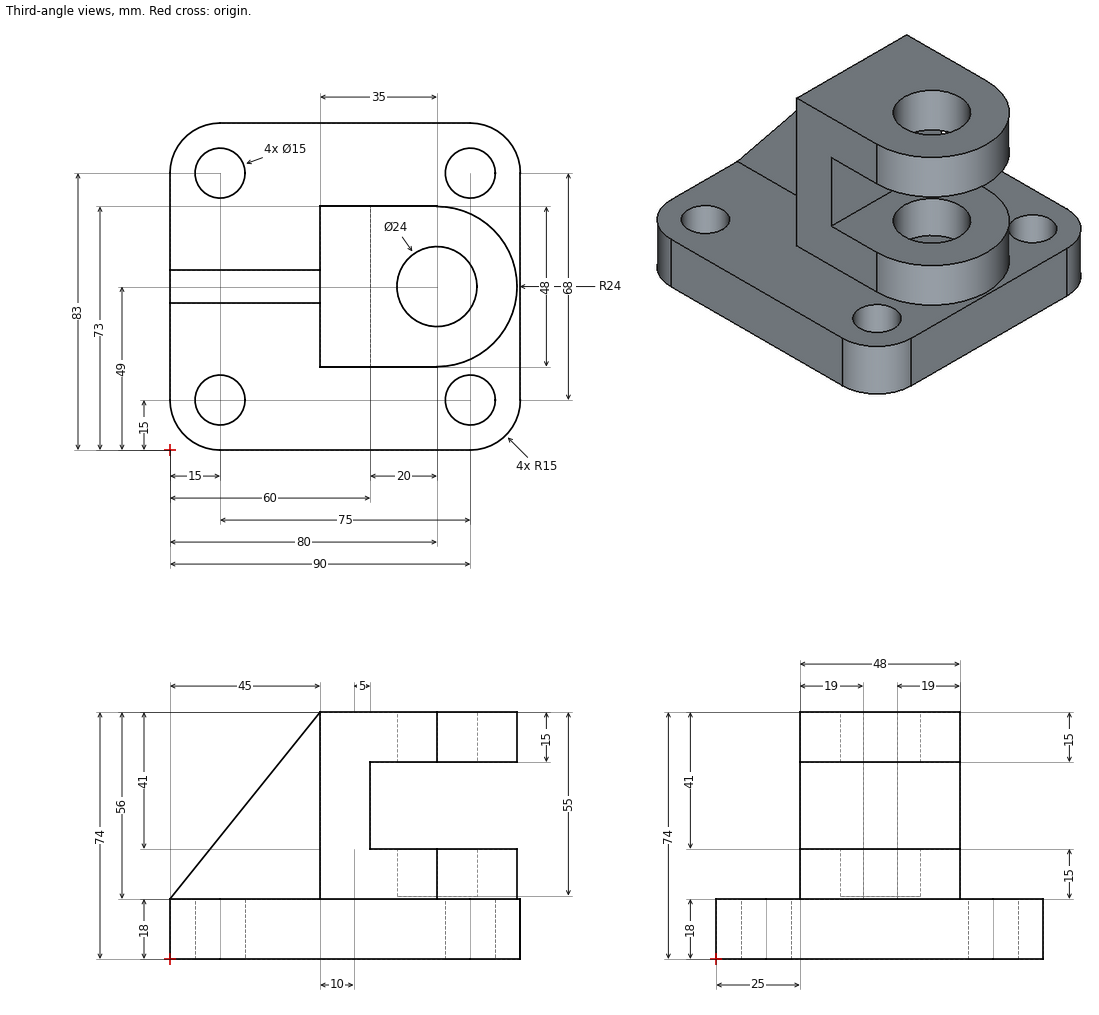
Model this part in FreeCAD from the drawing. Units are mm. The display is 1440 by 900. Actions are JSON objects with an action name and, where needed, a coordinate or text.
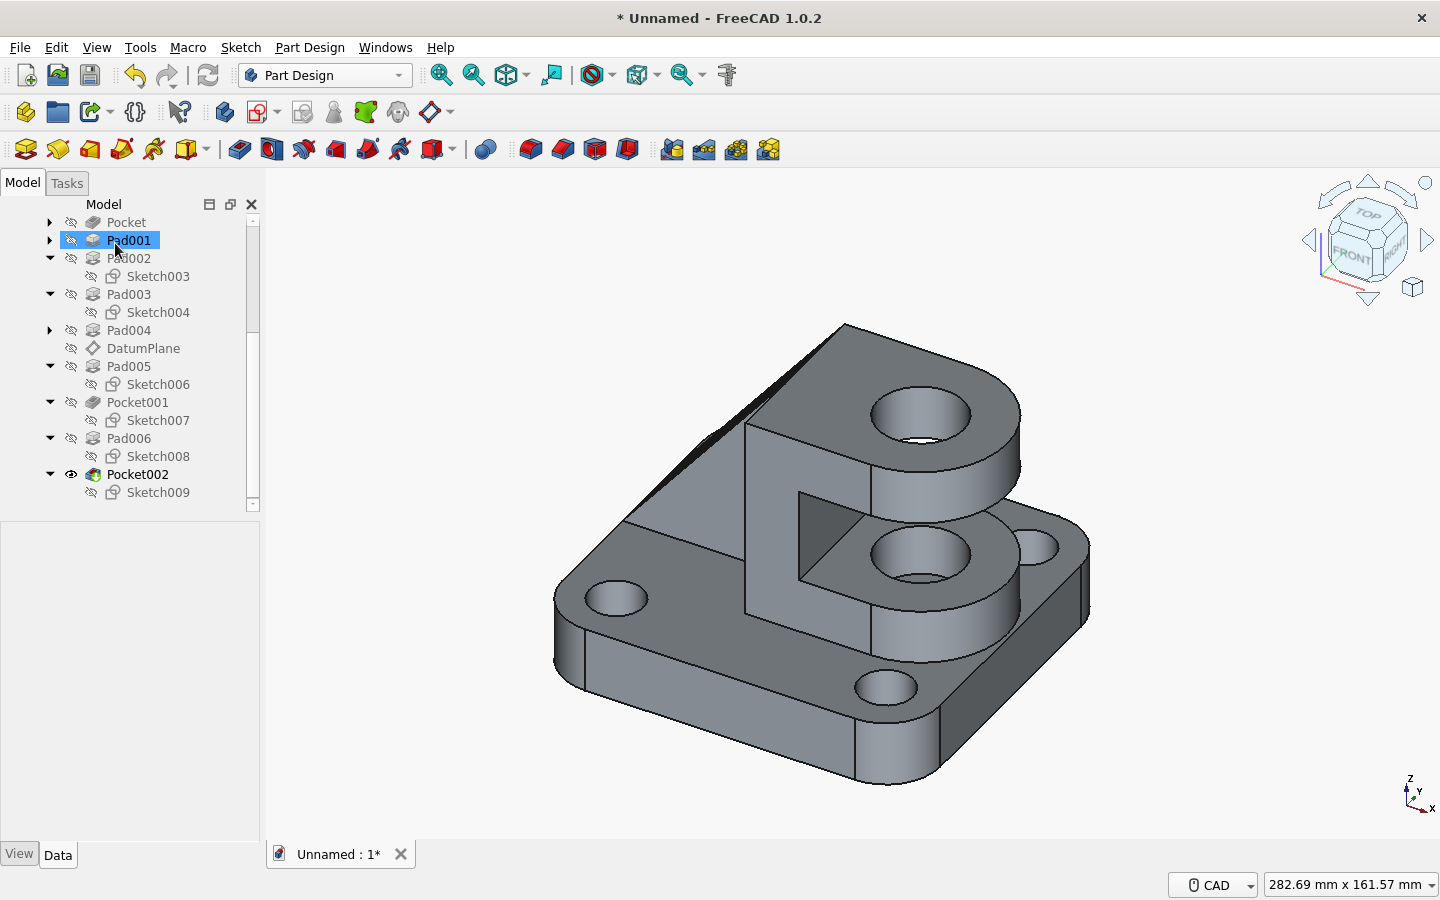
{"action": "key", "text": "4"}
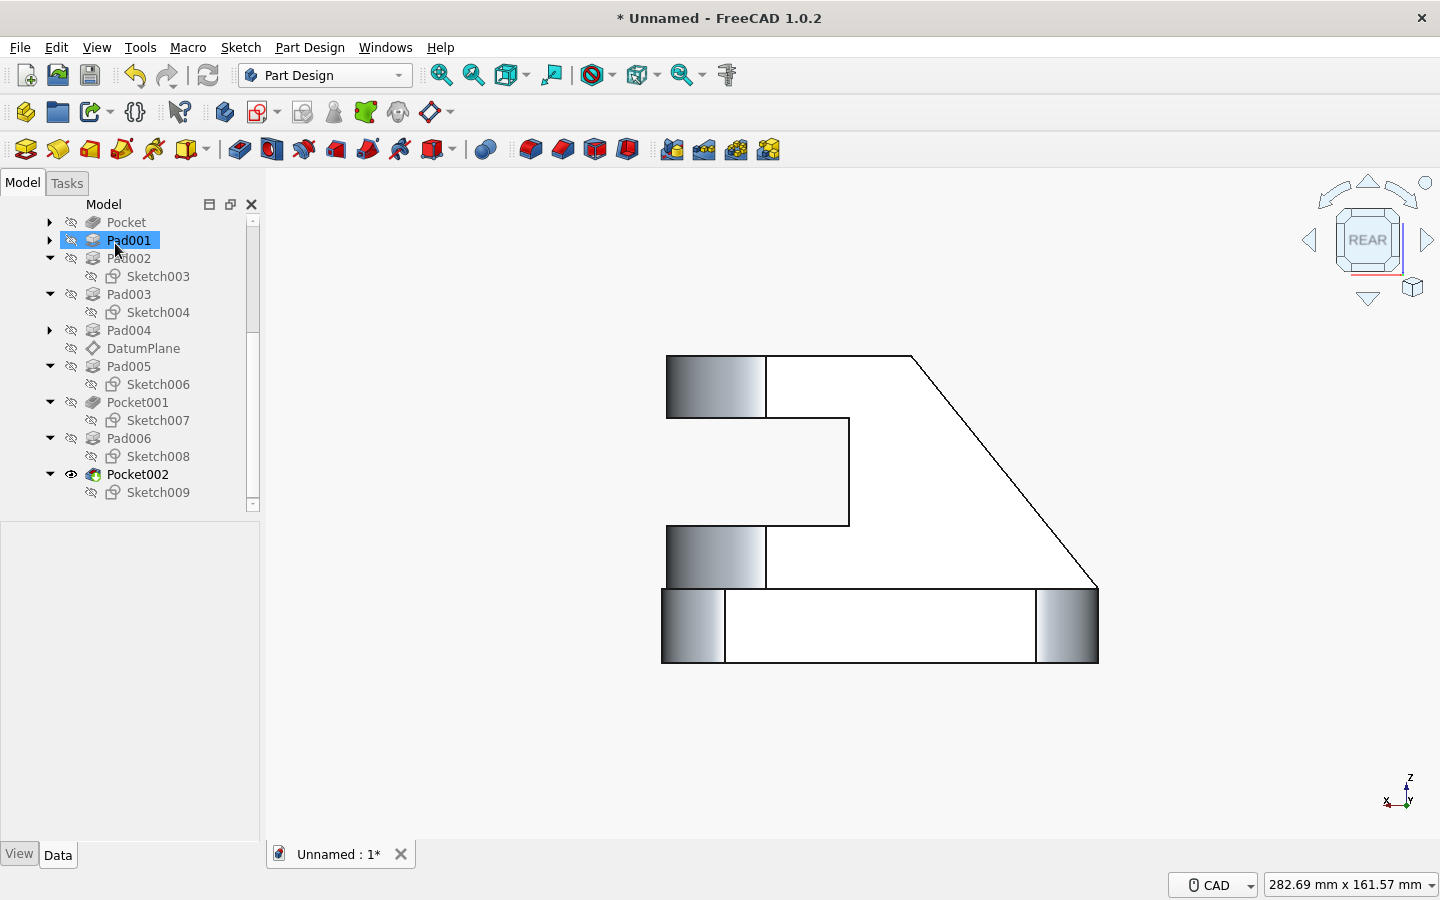
{"action": "left_click", "coordinate": [932, 505]}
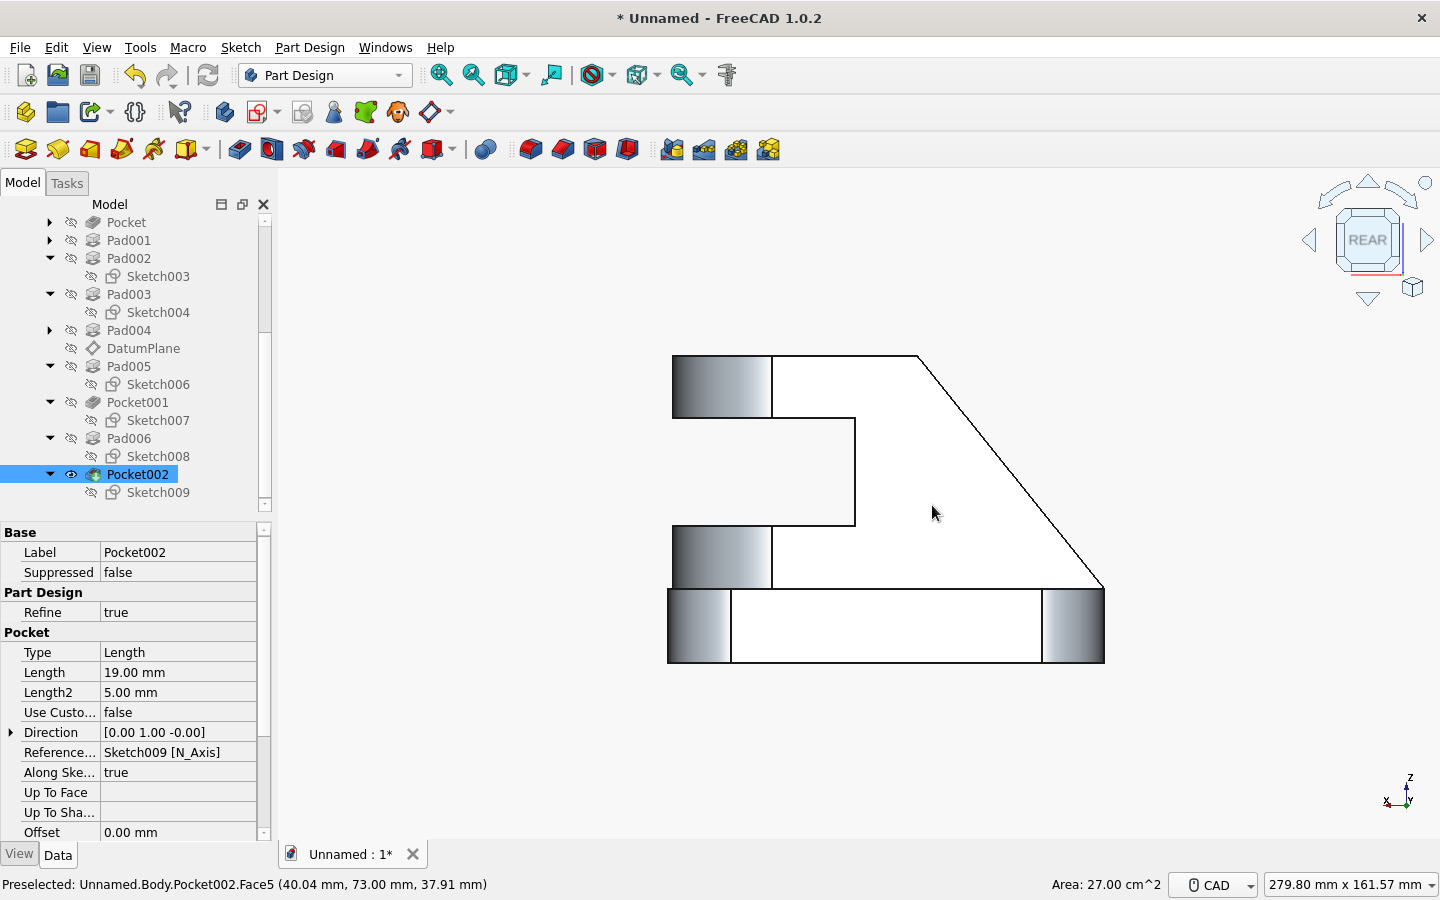
{"action": "left_click", "coordinate": [258, 112]}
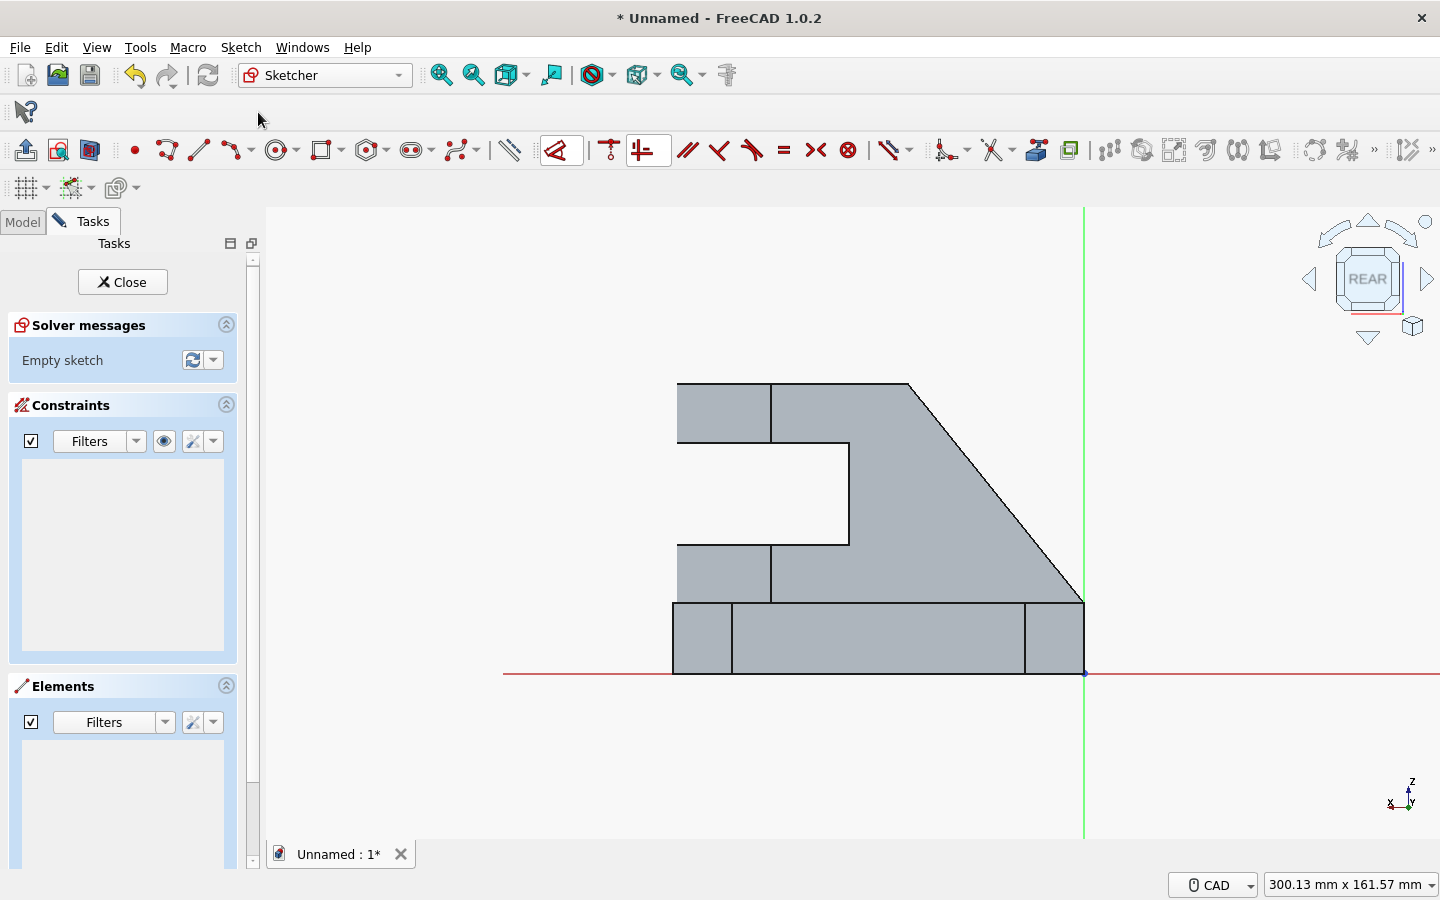
{"action": "left_click", "coordinate": [90, 150]}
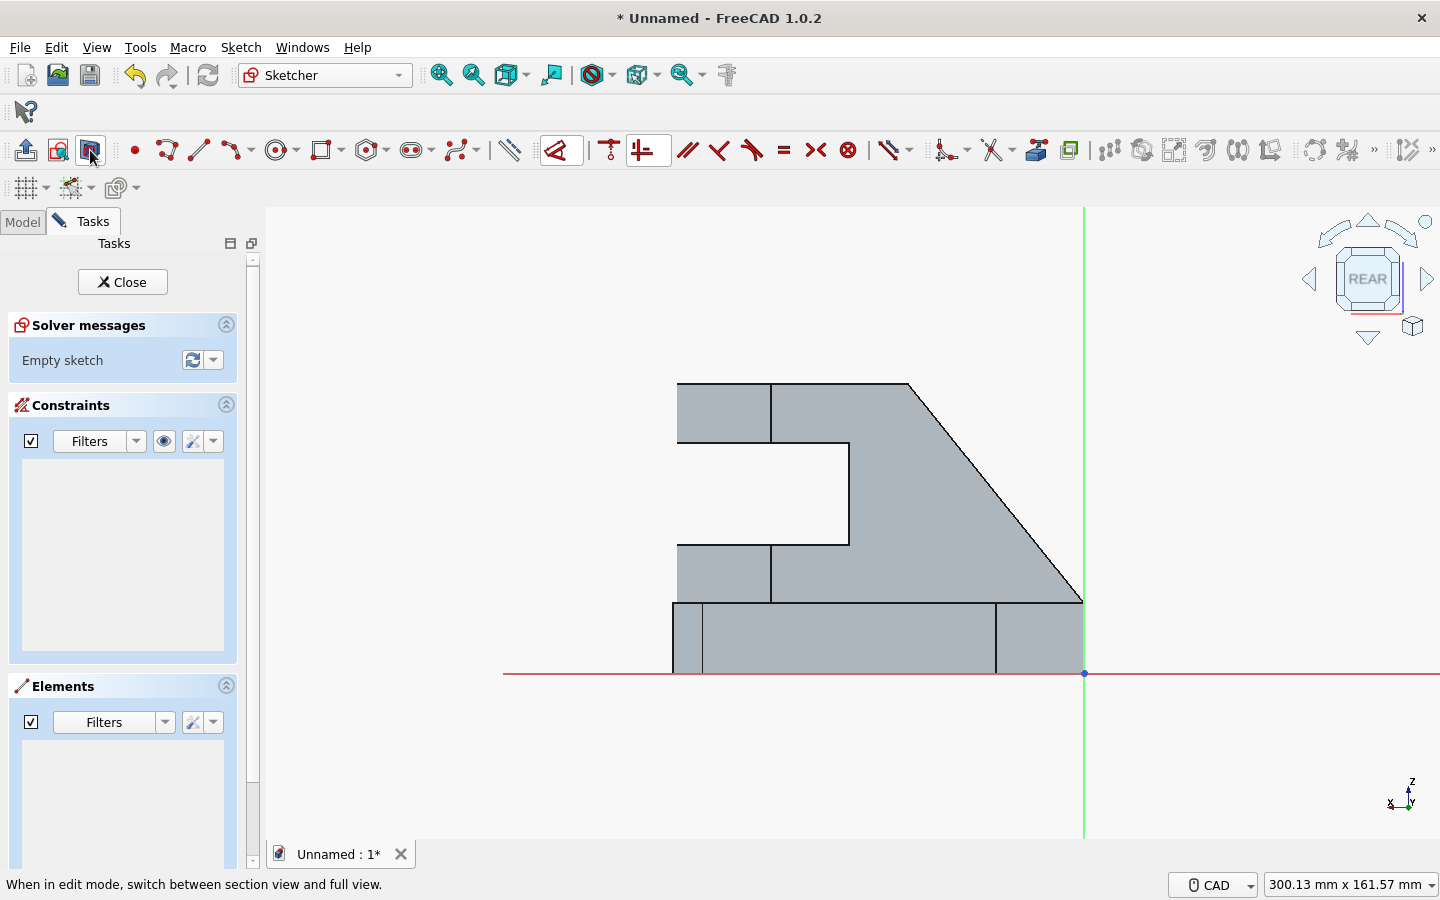
{"action": "scroll", "coordinate": [1275, 541], "scroll_direction": "up", "scroll_amount": 2}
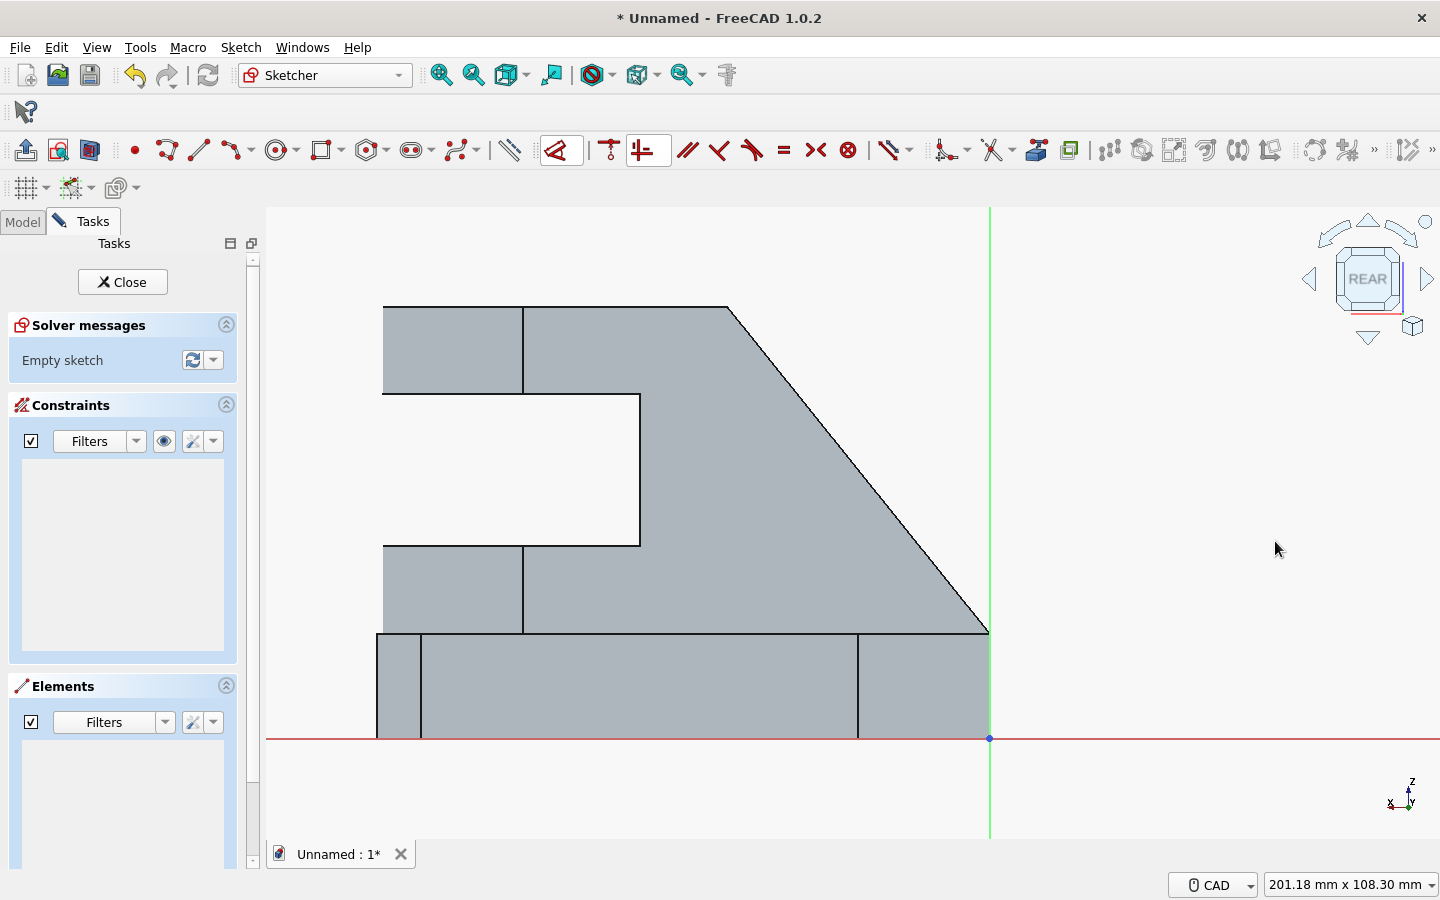
{"action": "left_click", "coordinate": [168, 150]}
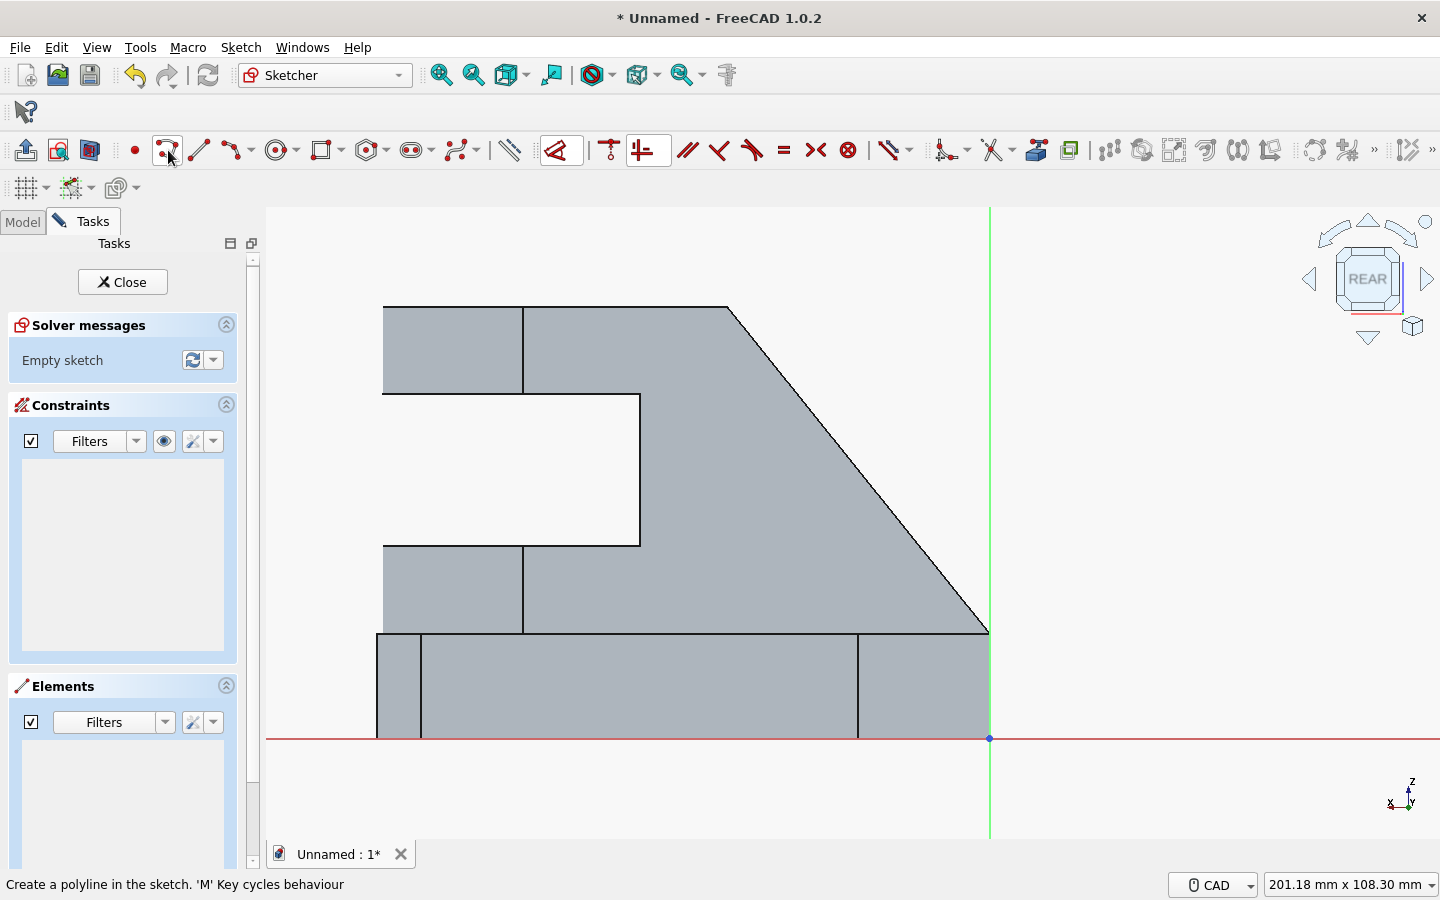
{"action": "left_click", "coordinate": [990, 634]}
{"action": "left_click", "coordinate": [727, 307]}
{"action": "left_click", "coordinate": [727, 634]}
{"action": "left_click", "coordinate": [990, 635]}
{"action": "key", "text": "Escape"}
{"action": "key", "text": "Escape"}